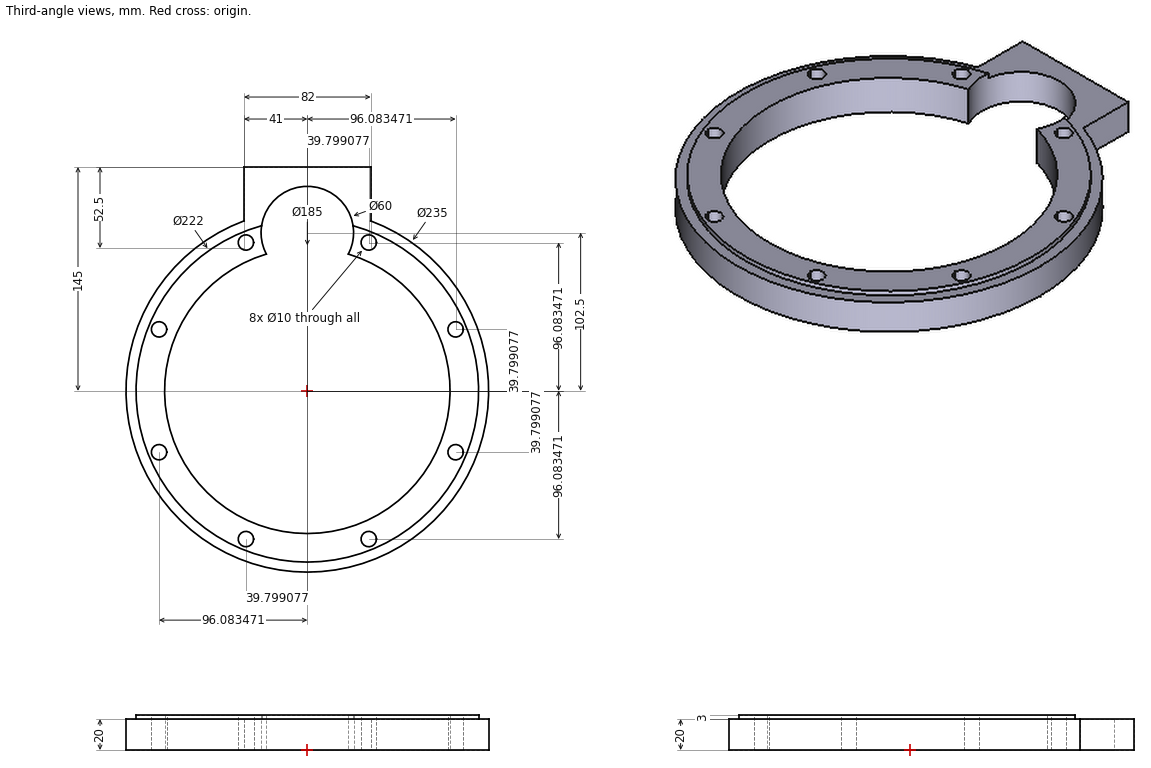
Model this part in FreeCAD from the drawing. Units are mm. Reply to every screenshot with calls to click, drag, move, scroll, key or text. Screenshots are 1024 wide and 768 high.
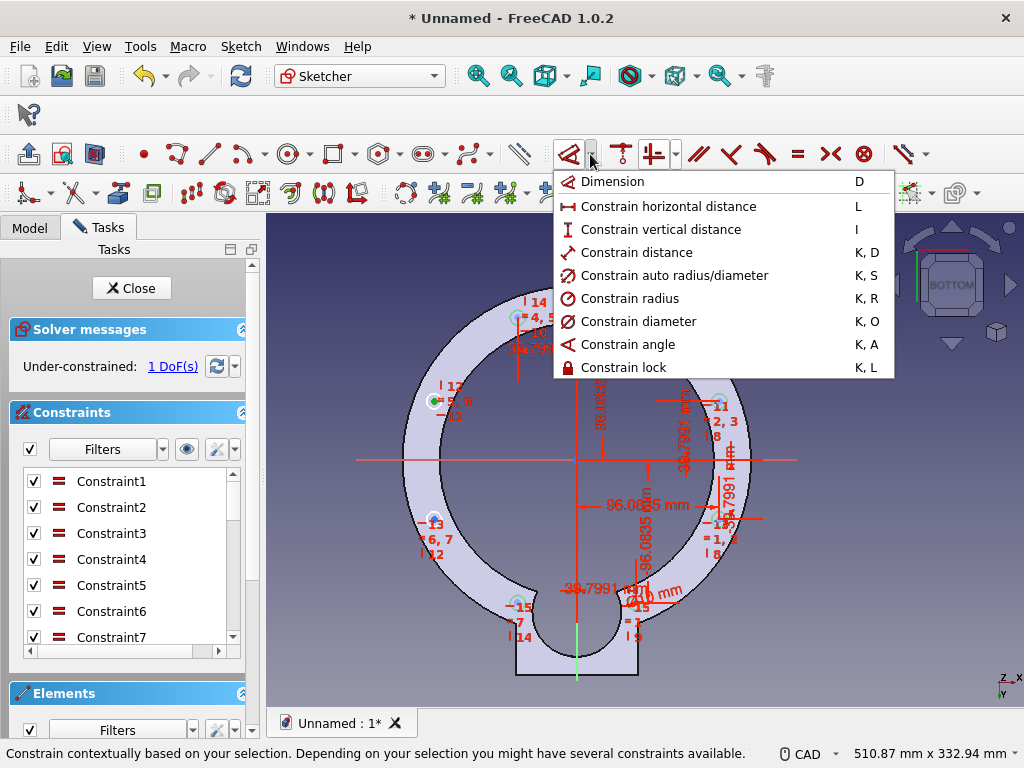
click(724, 206)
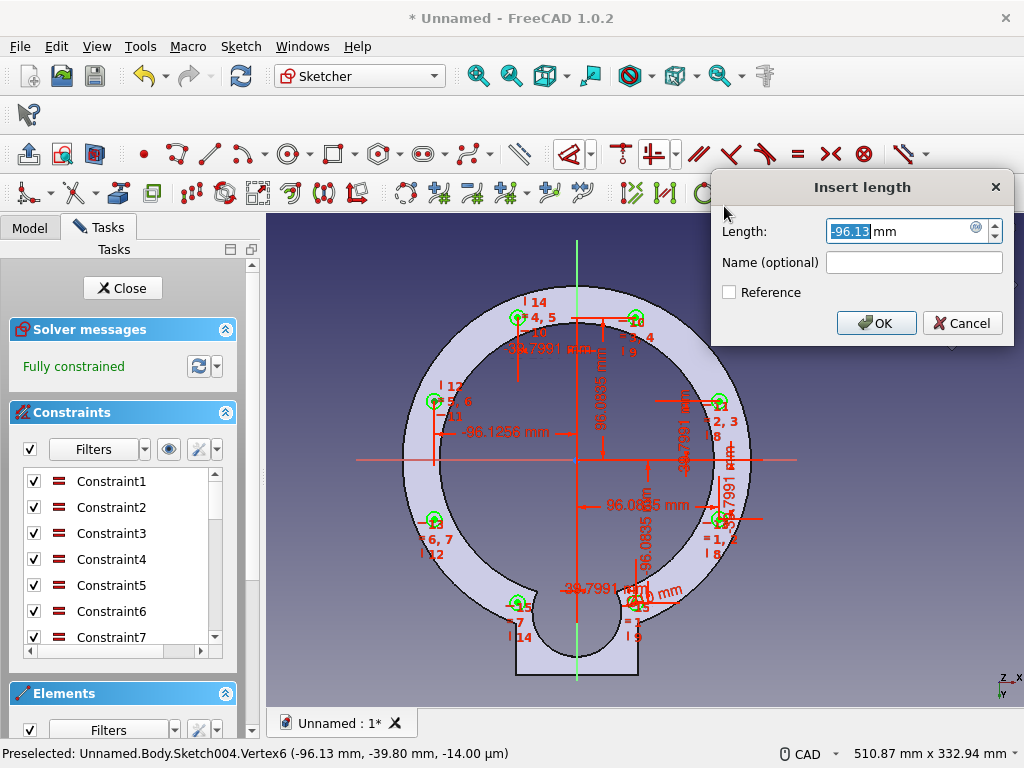
text(-96.083471)
key(Return)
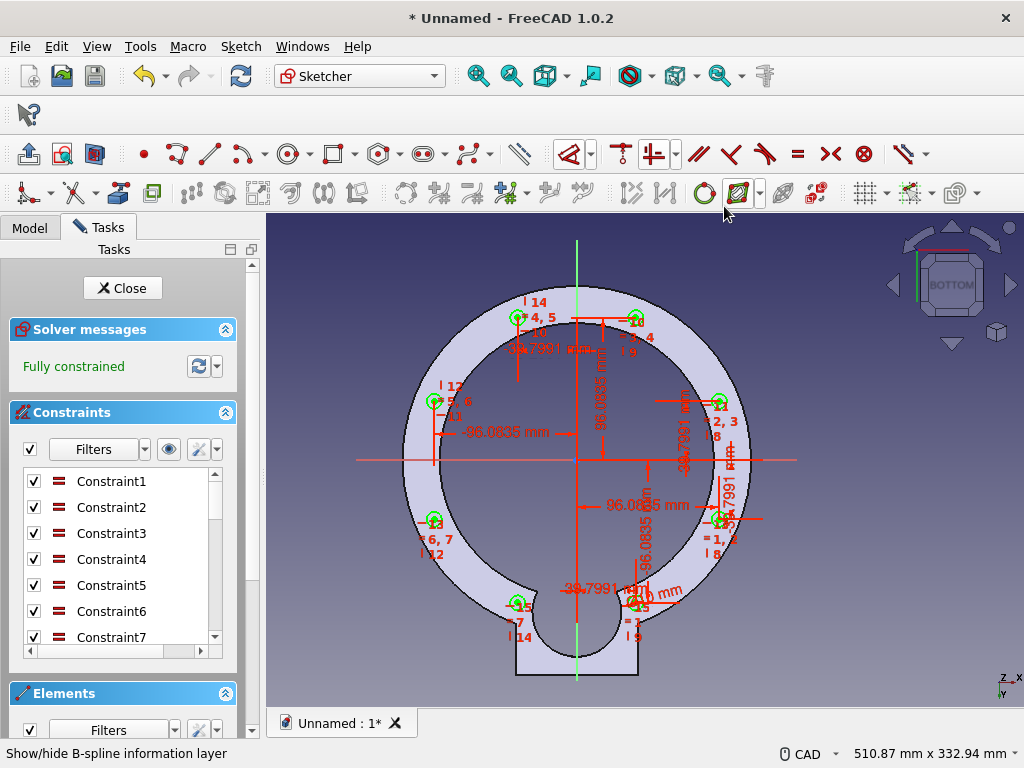
click(123, 288)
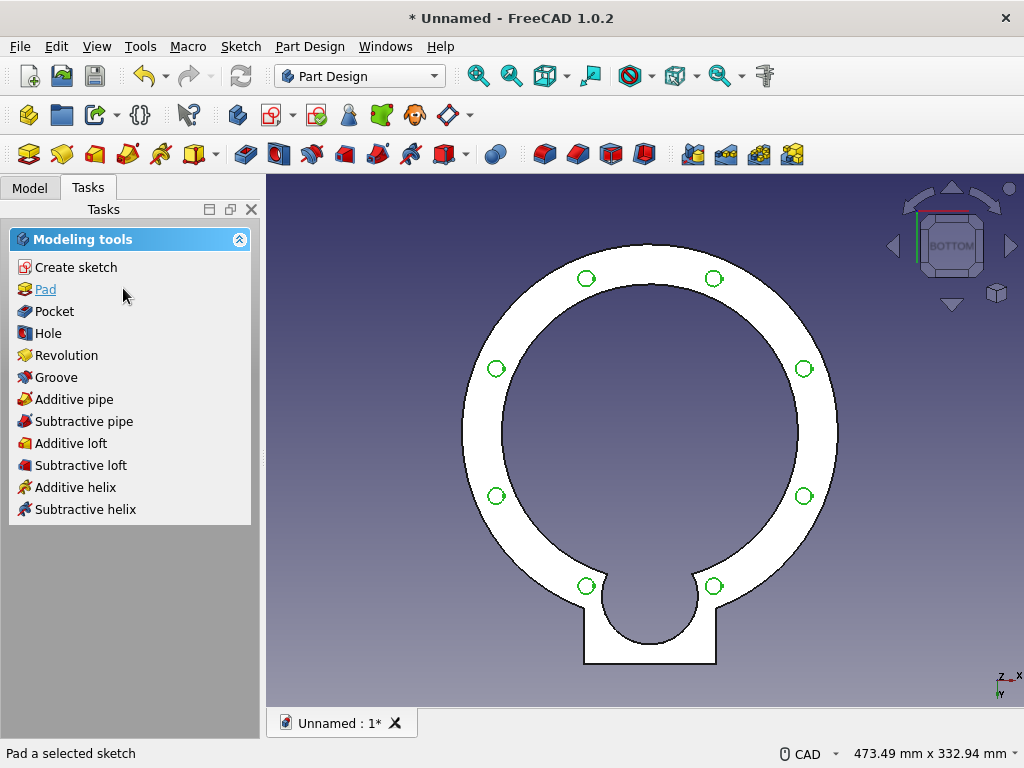
click(279, 154)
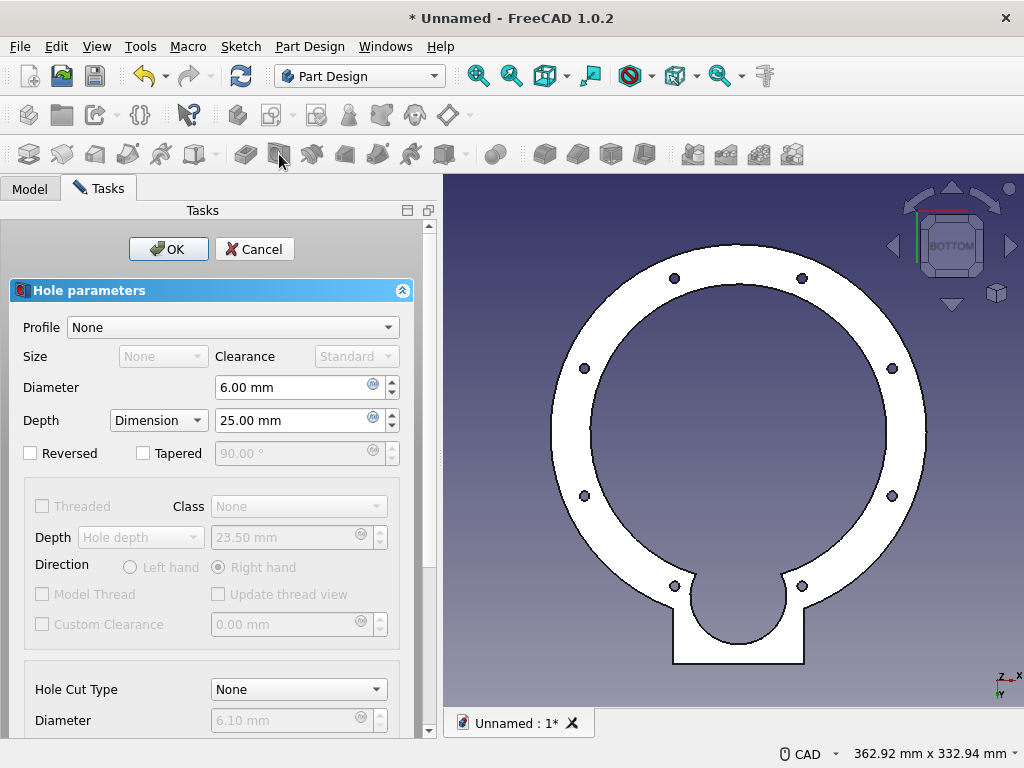
triple_click(300, 388)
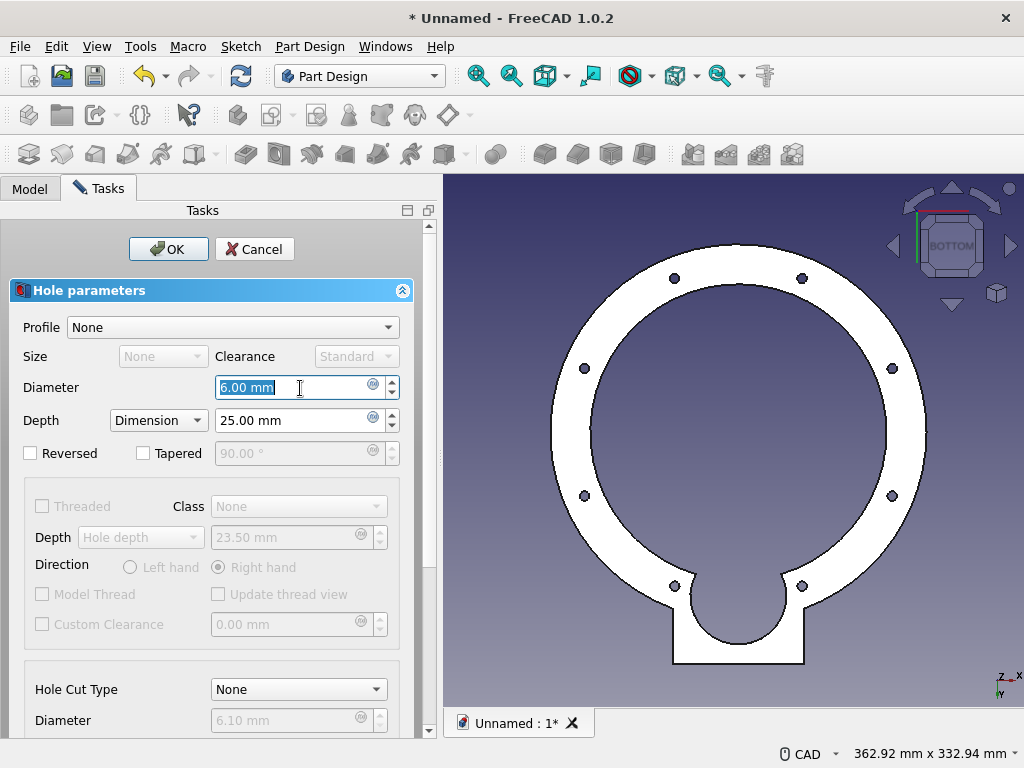
text(10)
key(Tab)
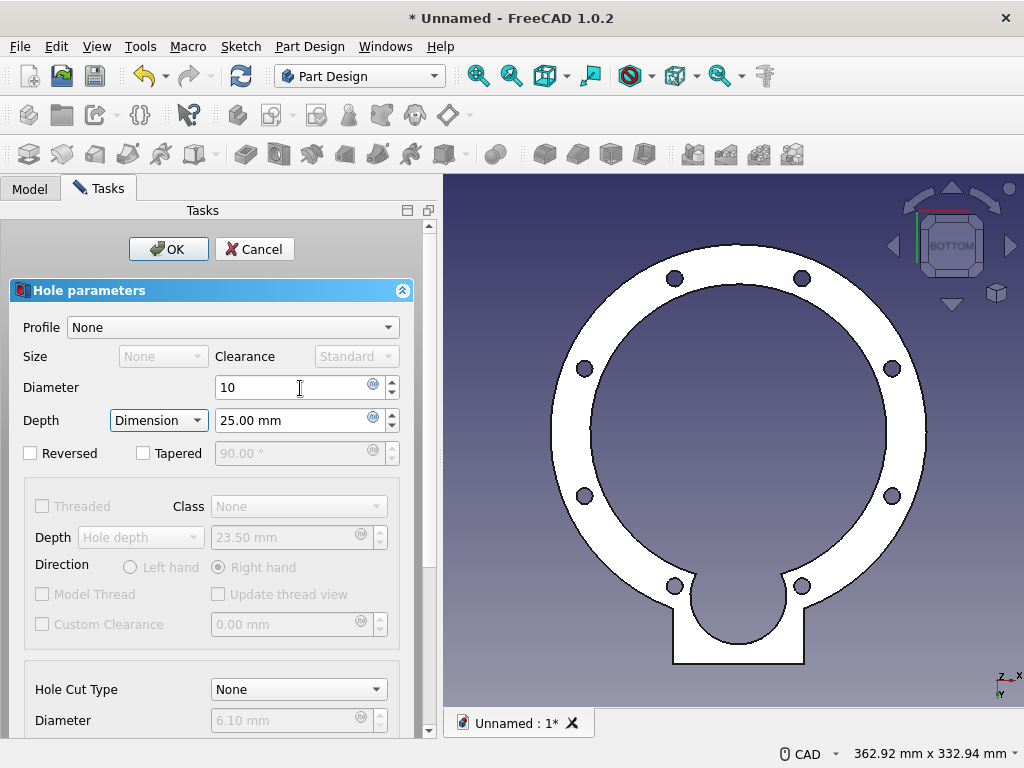
click(160, 420)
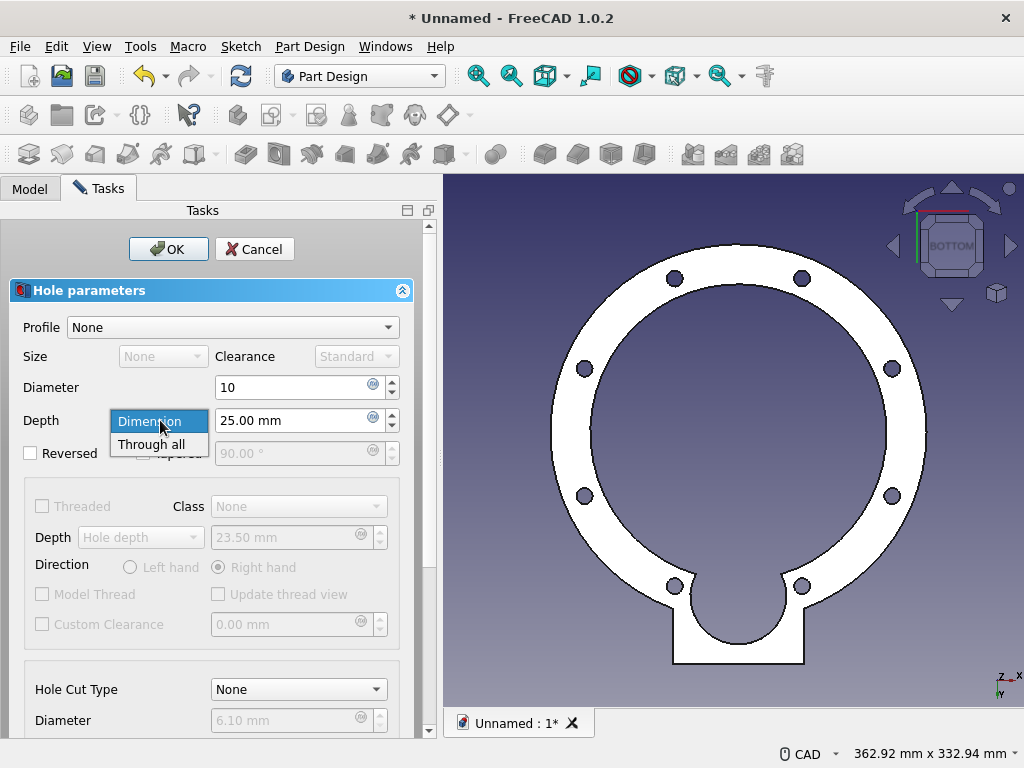
click(158, 444)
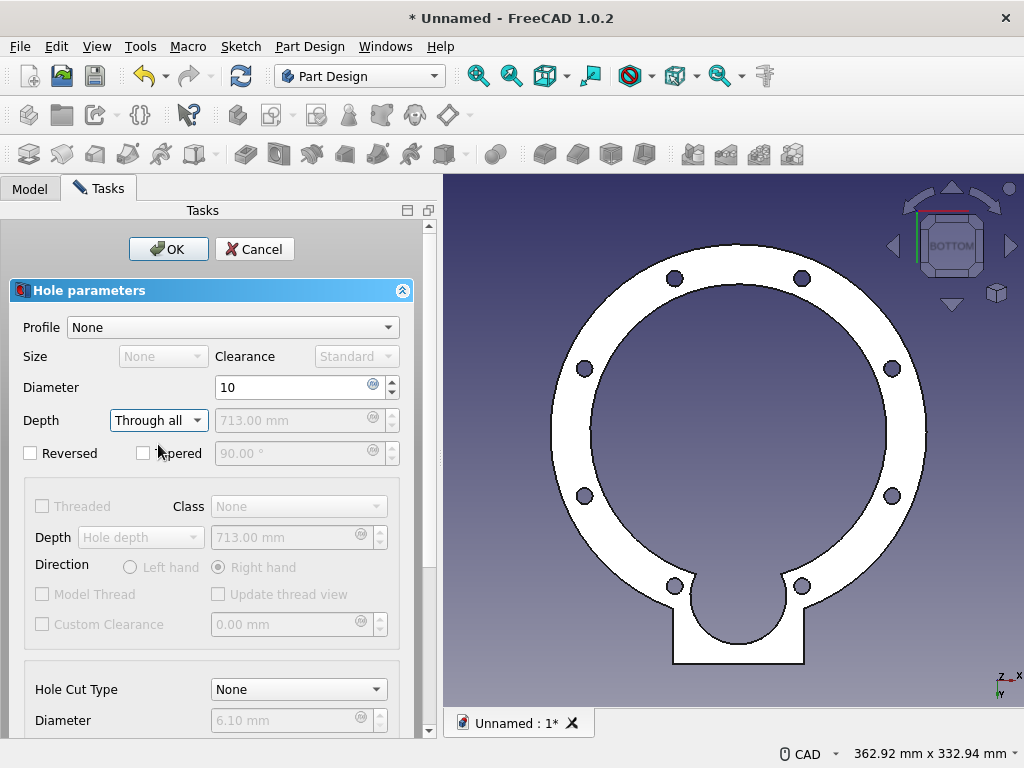
click(169, 249)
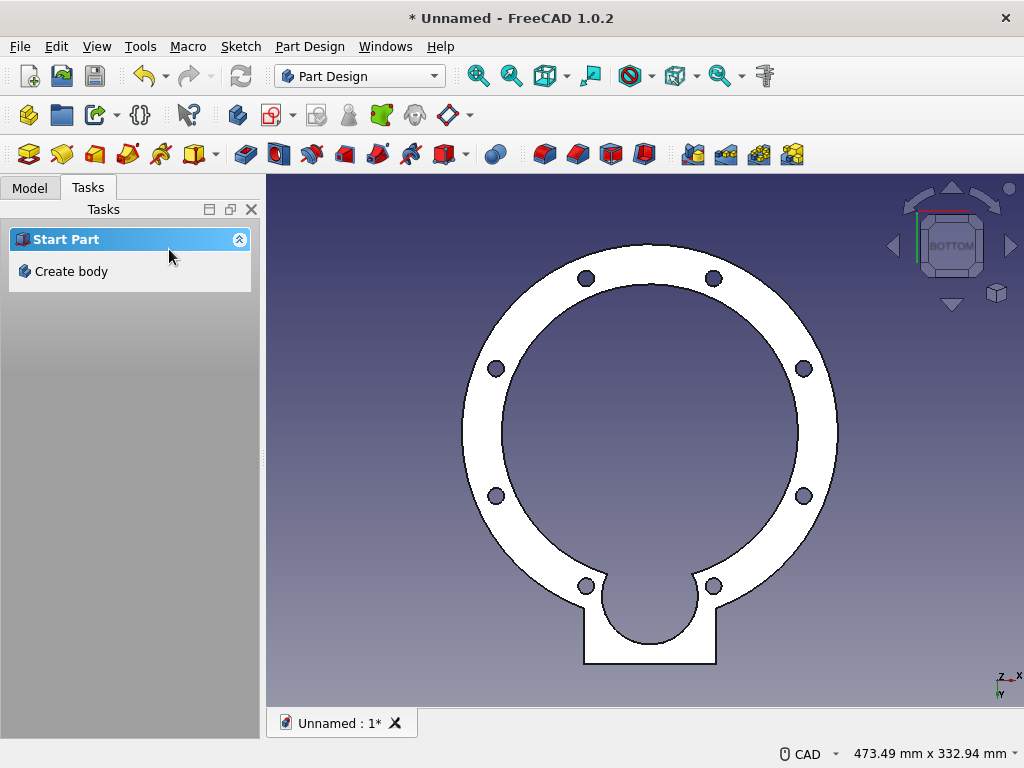
key(0)